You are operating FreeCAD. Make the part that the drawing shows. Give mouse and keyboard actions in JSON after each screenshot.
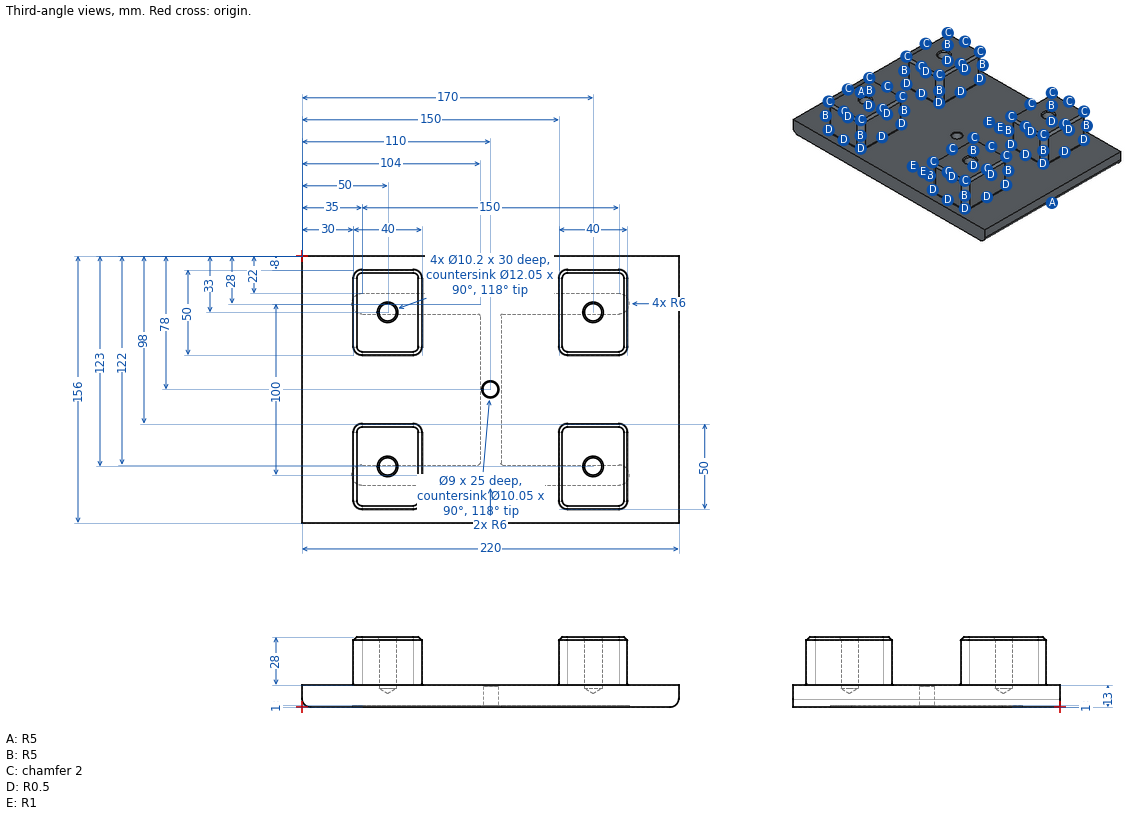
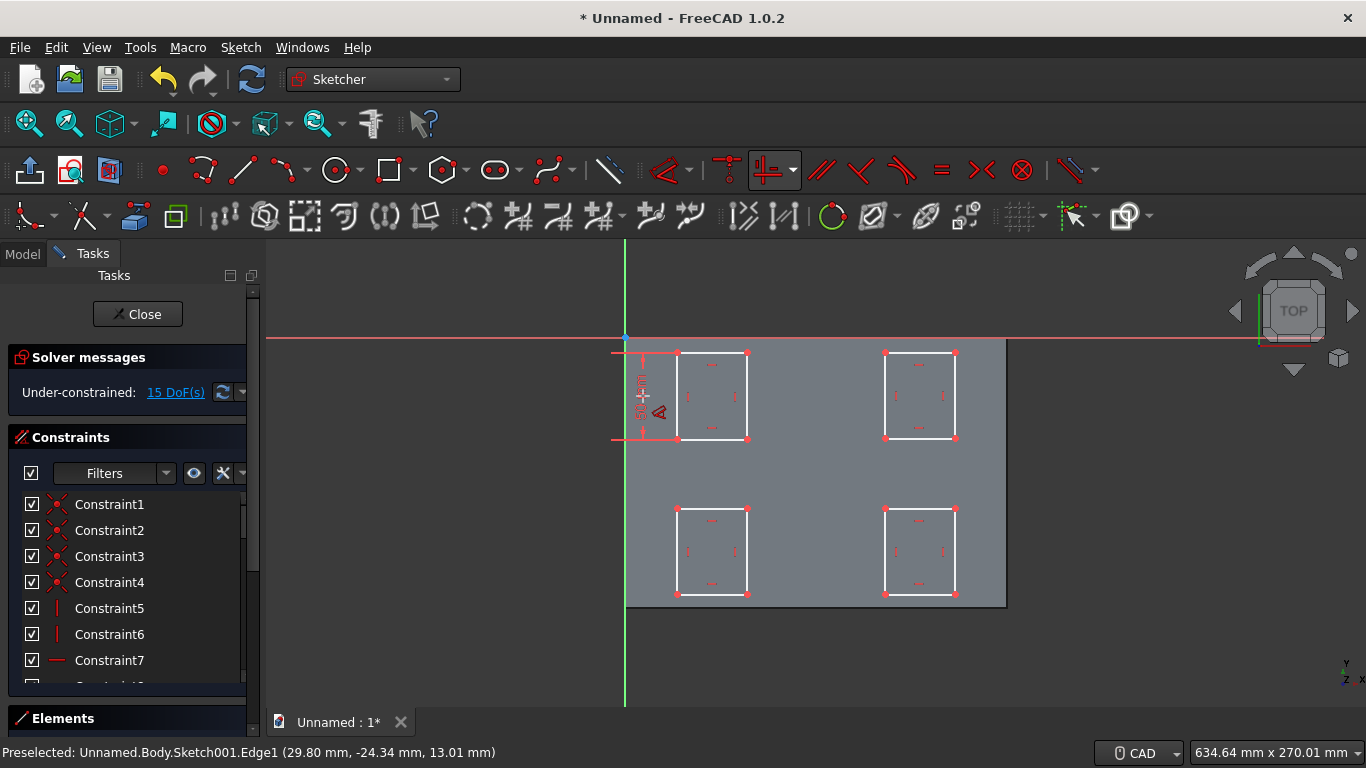
{"action": "left_click", "coordinate": [698, 440]}
{"action": "left_click", "coordinate": [728, 406]}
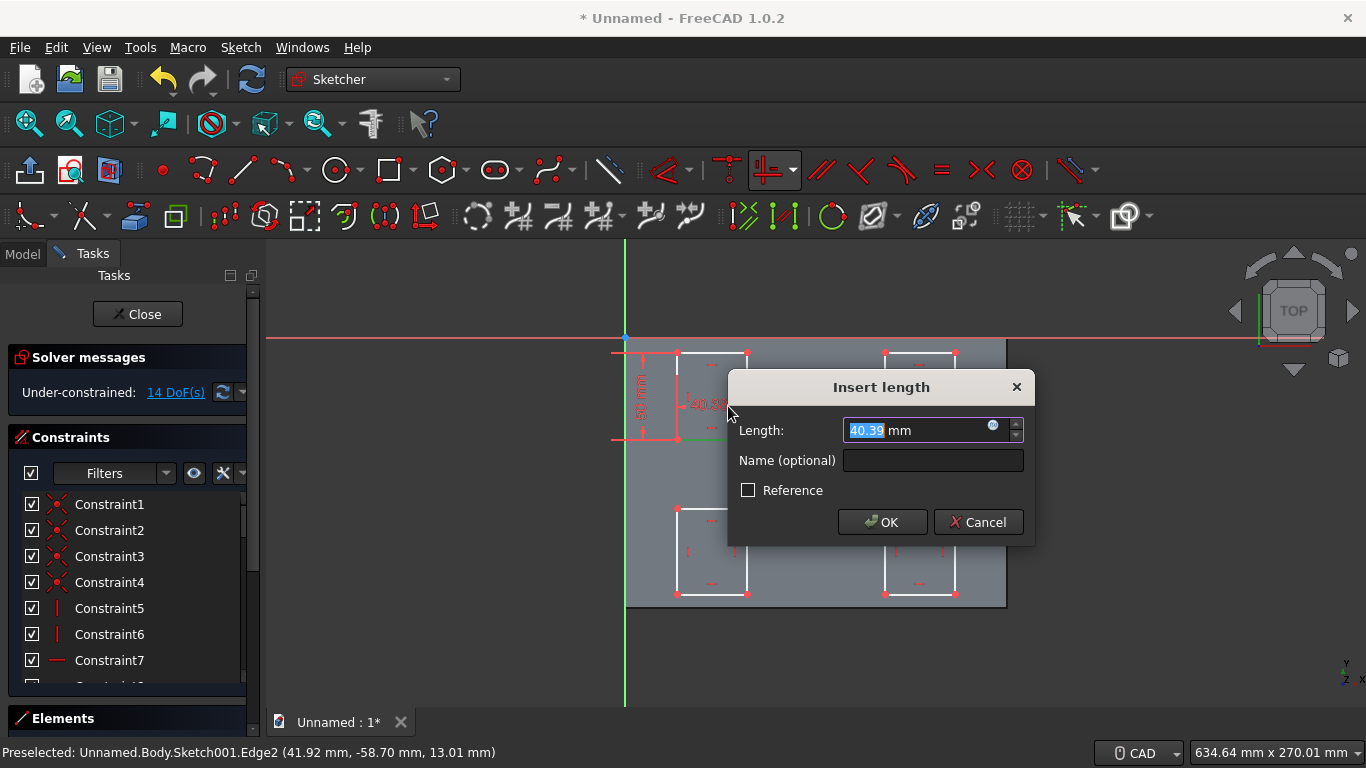
{"action": "type", "text": "40"}
{"action": "key", "text": "Return"}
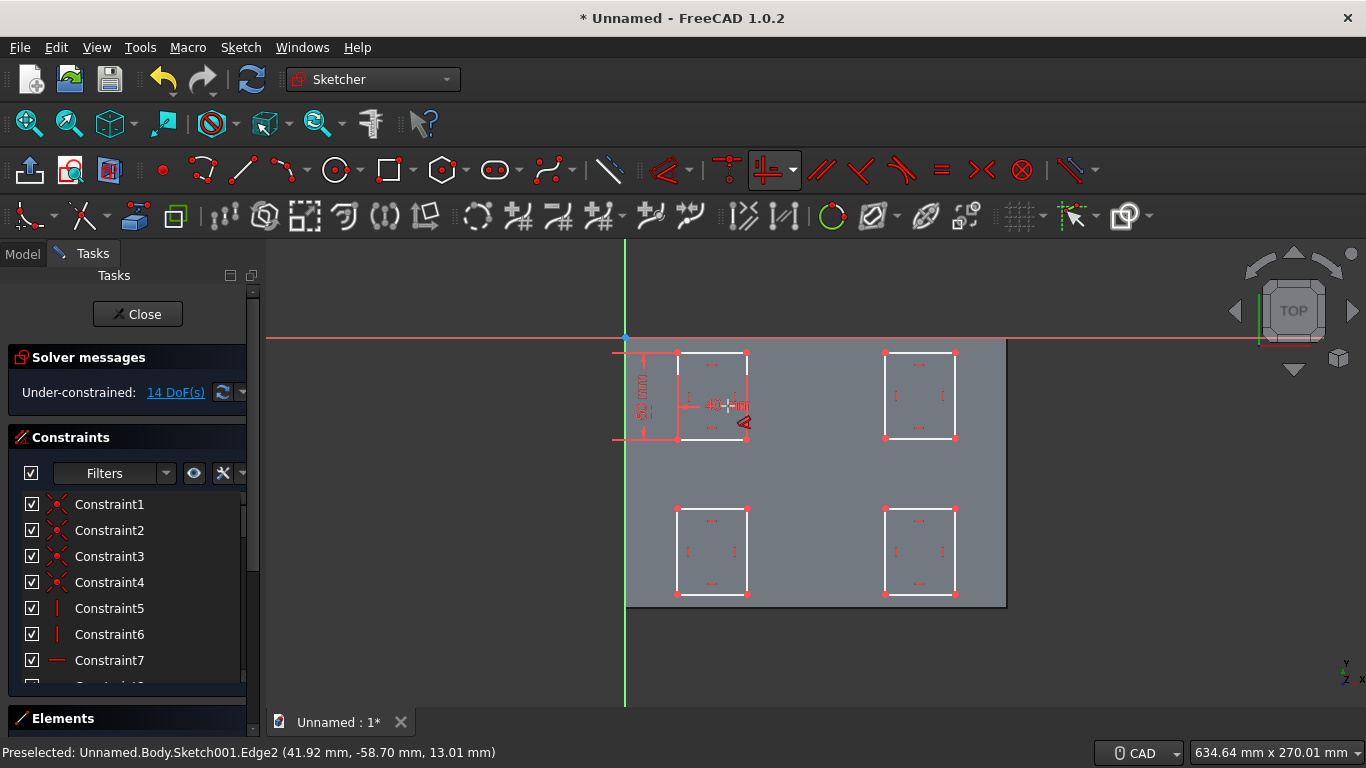
{"action": "left_click", "coordinate": [885, 379]}
{"action": "left_click", "coordinate": [919, 396]}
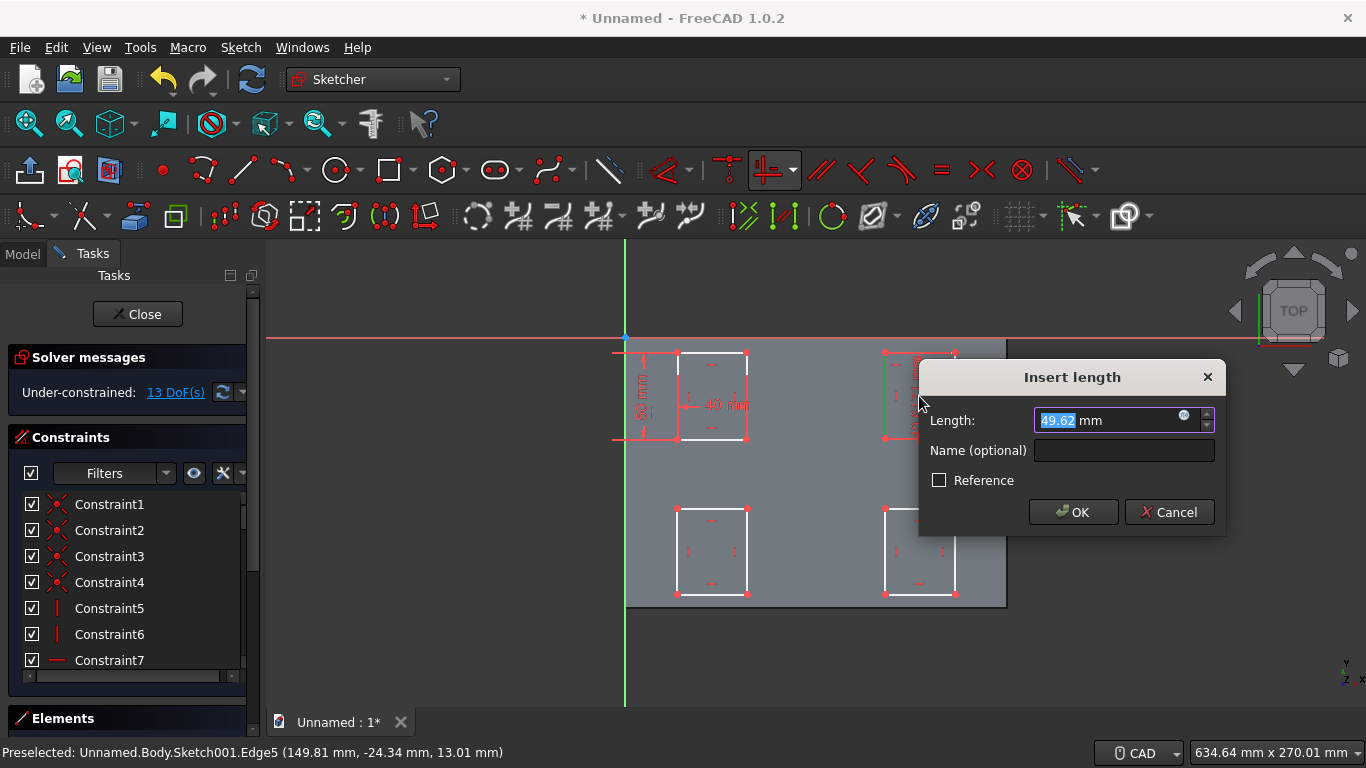
{"action": "type", "text": "50"}
{"action": "key", "text": "Return"}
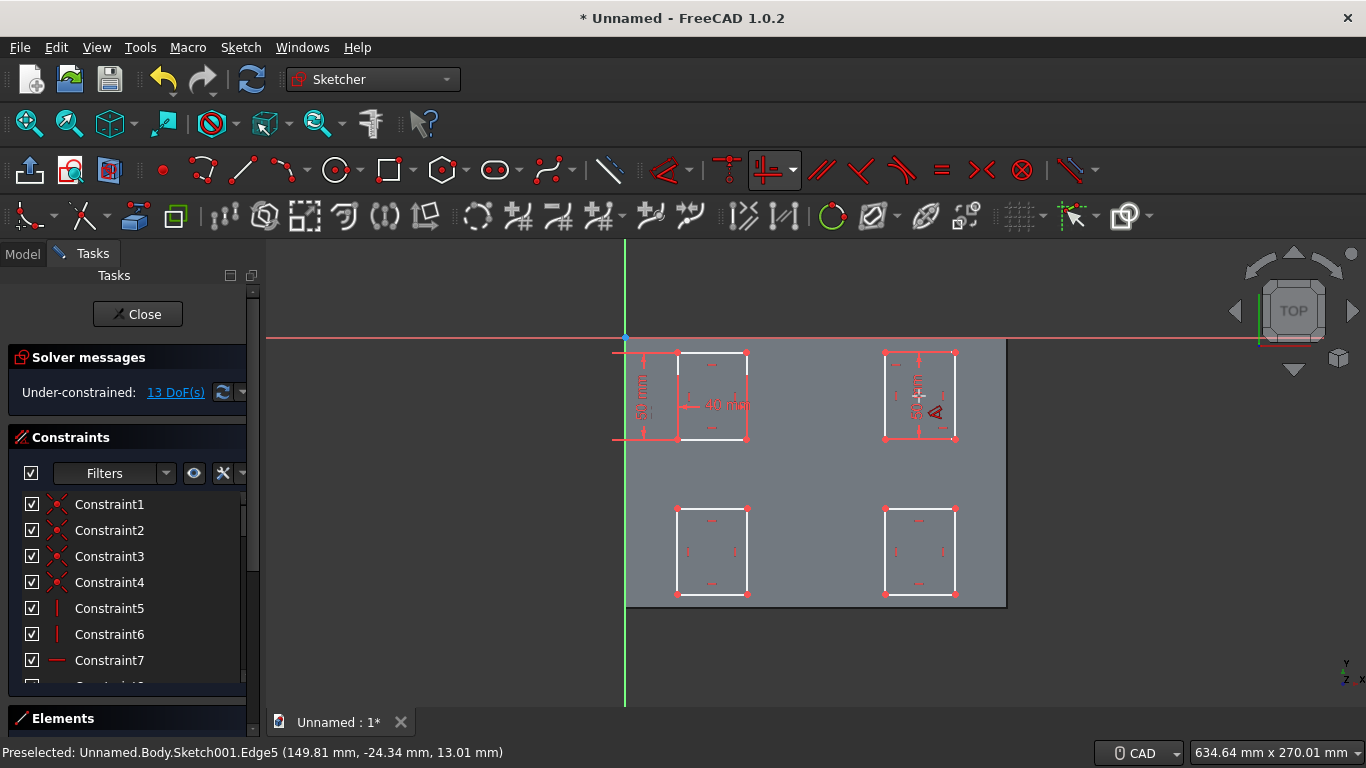
{"action": "left_click", "coordinate": [906, 439]}
{"action": "left_click", "coordinate": [920, 473]}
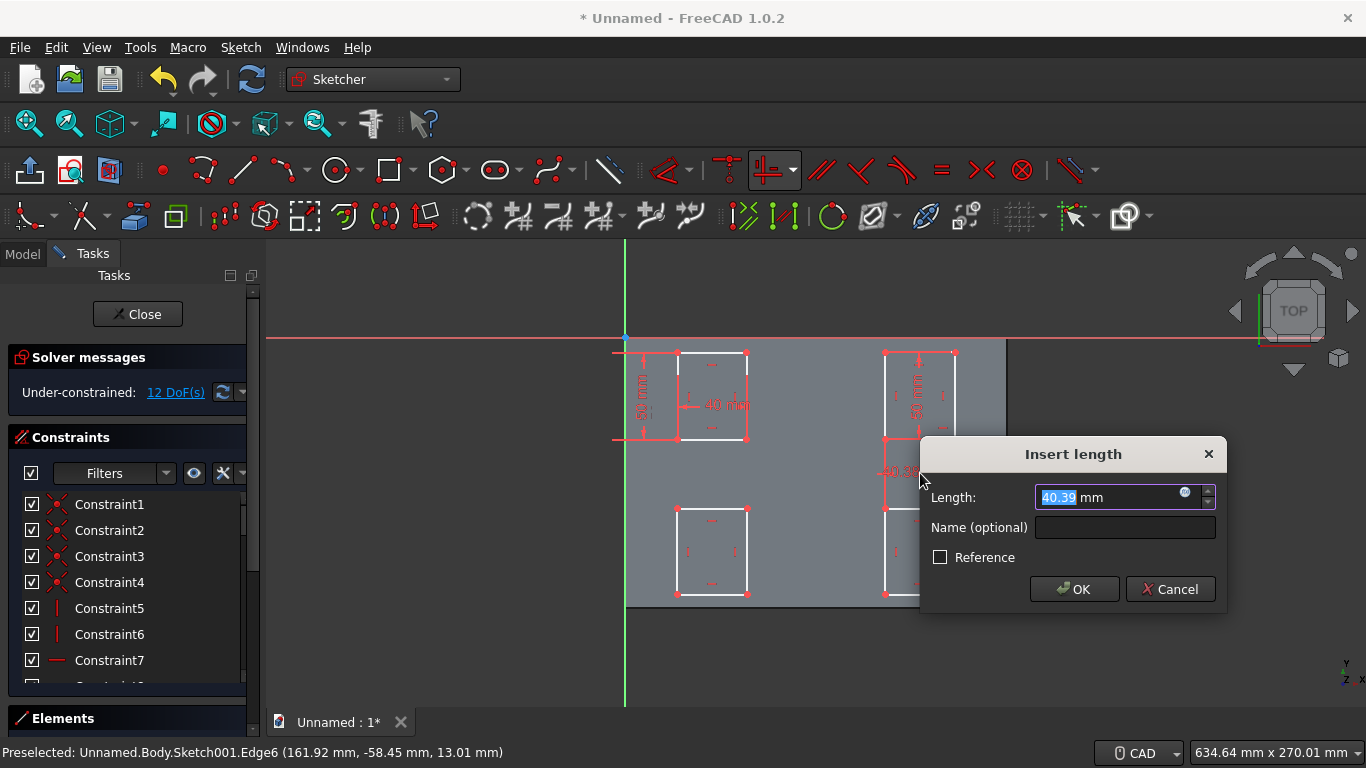
{"action": "type", "text": "40"}
{"action": "key", "text": "Return"}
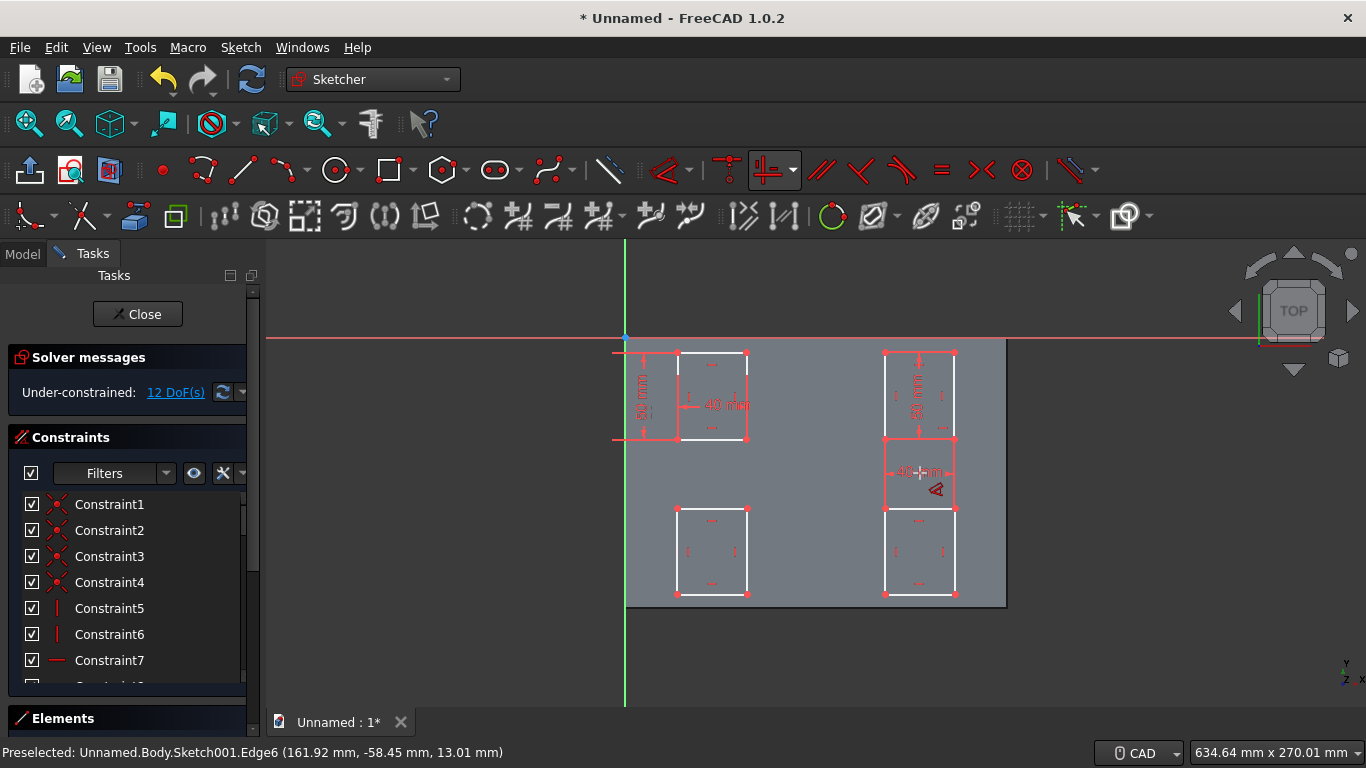
{"action": "left_click", "coordinate": [885, 535]}
{"action": "left_click", "coordinate": [919, 552]}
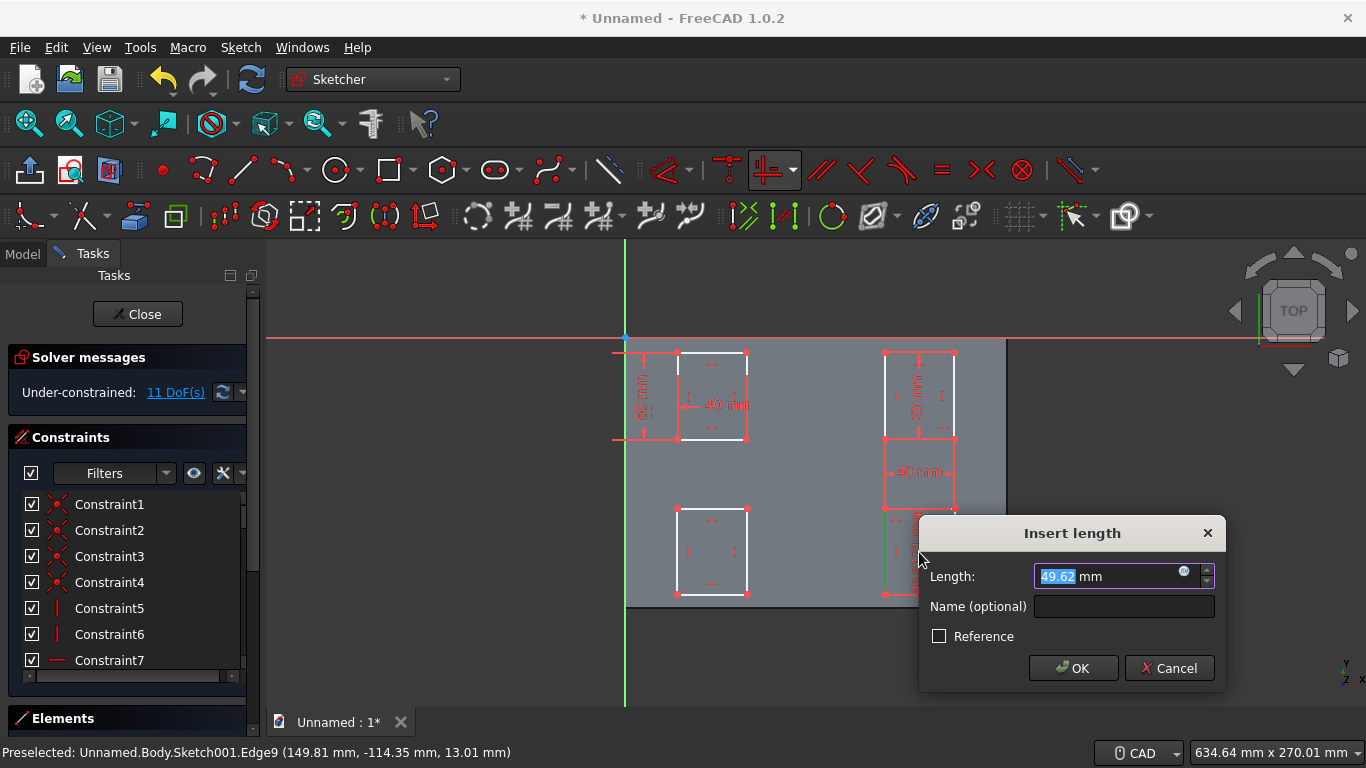
{"action": "type", "text": "50"}
{"action": "key", "text": "Return"}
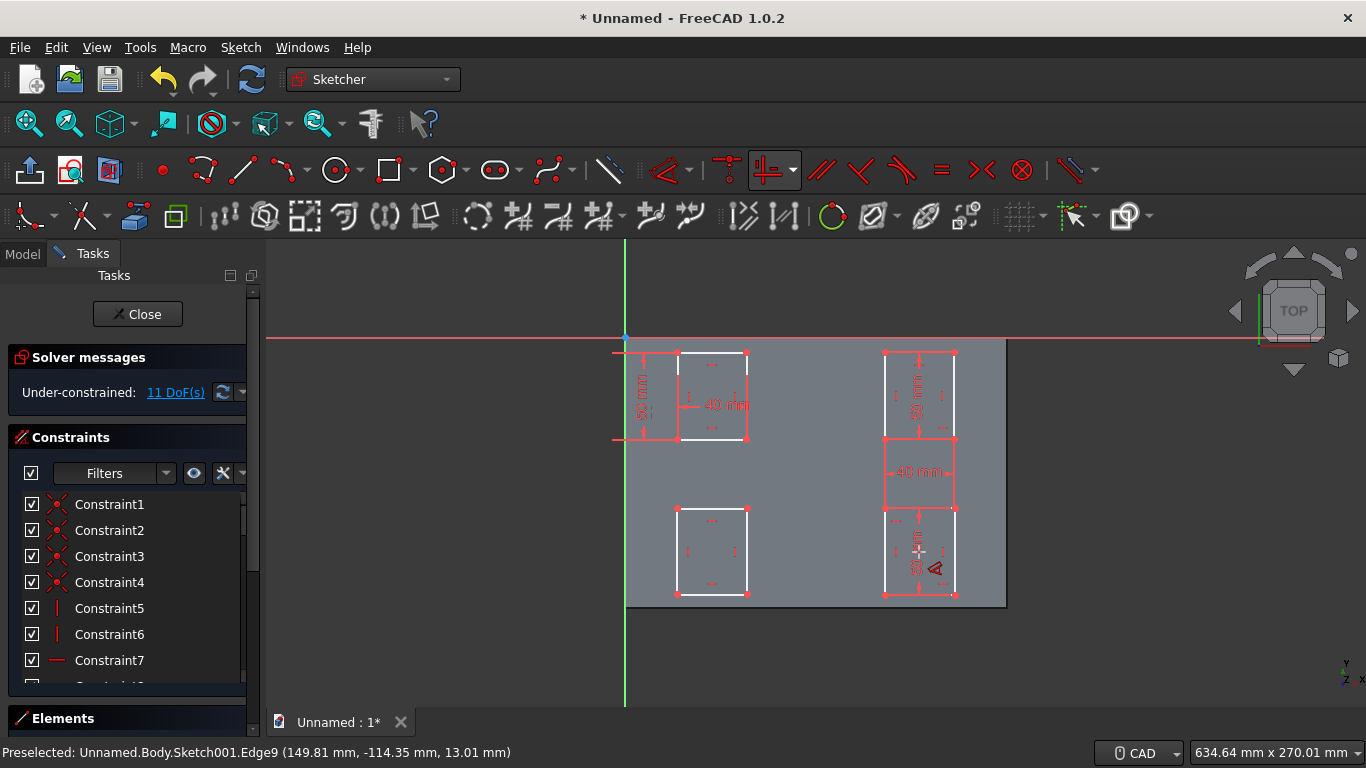
{"action": "left_click", "coordinate": [906, 595]}
{"action": "left_click", "coordinate": [920, 629]}